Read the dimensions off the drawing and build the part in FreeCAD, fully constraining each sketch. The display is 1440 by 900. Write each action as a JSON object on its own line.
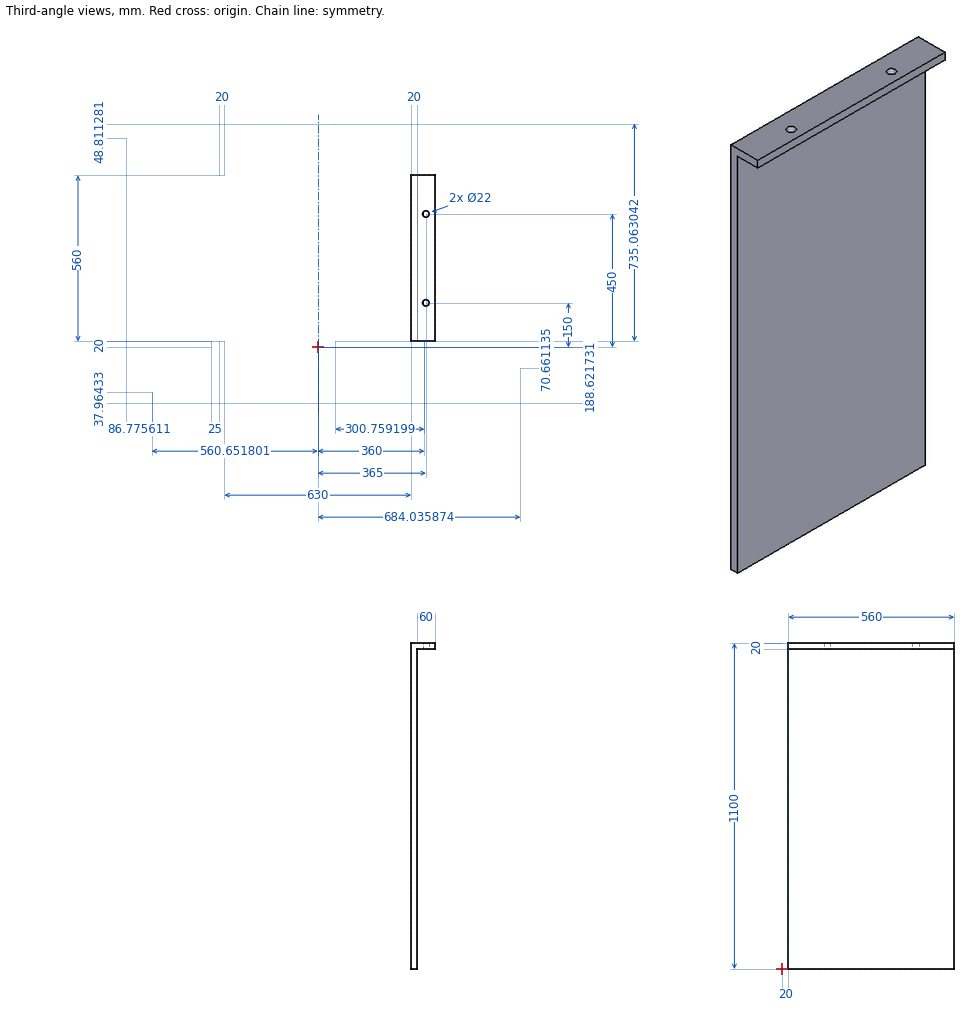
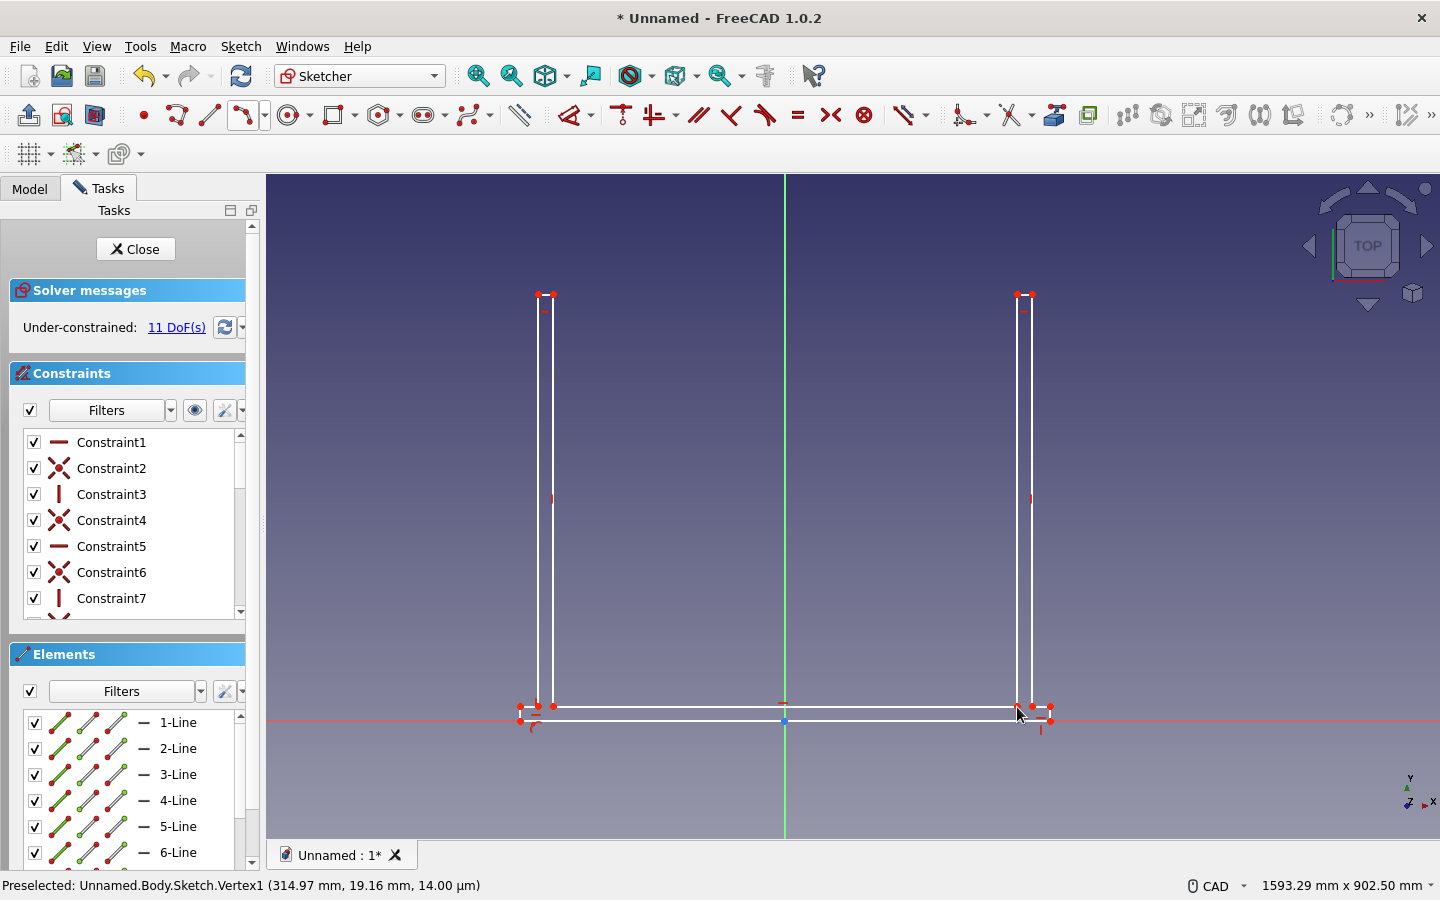
{"action": "left_click", "coordinate": [520, 707]}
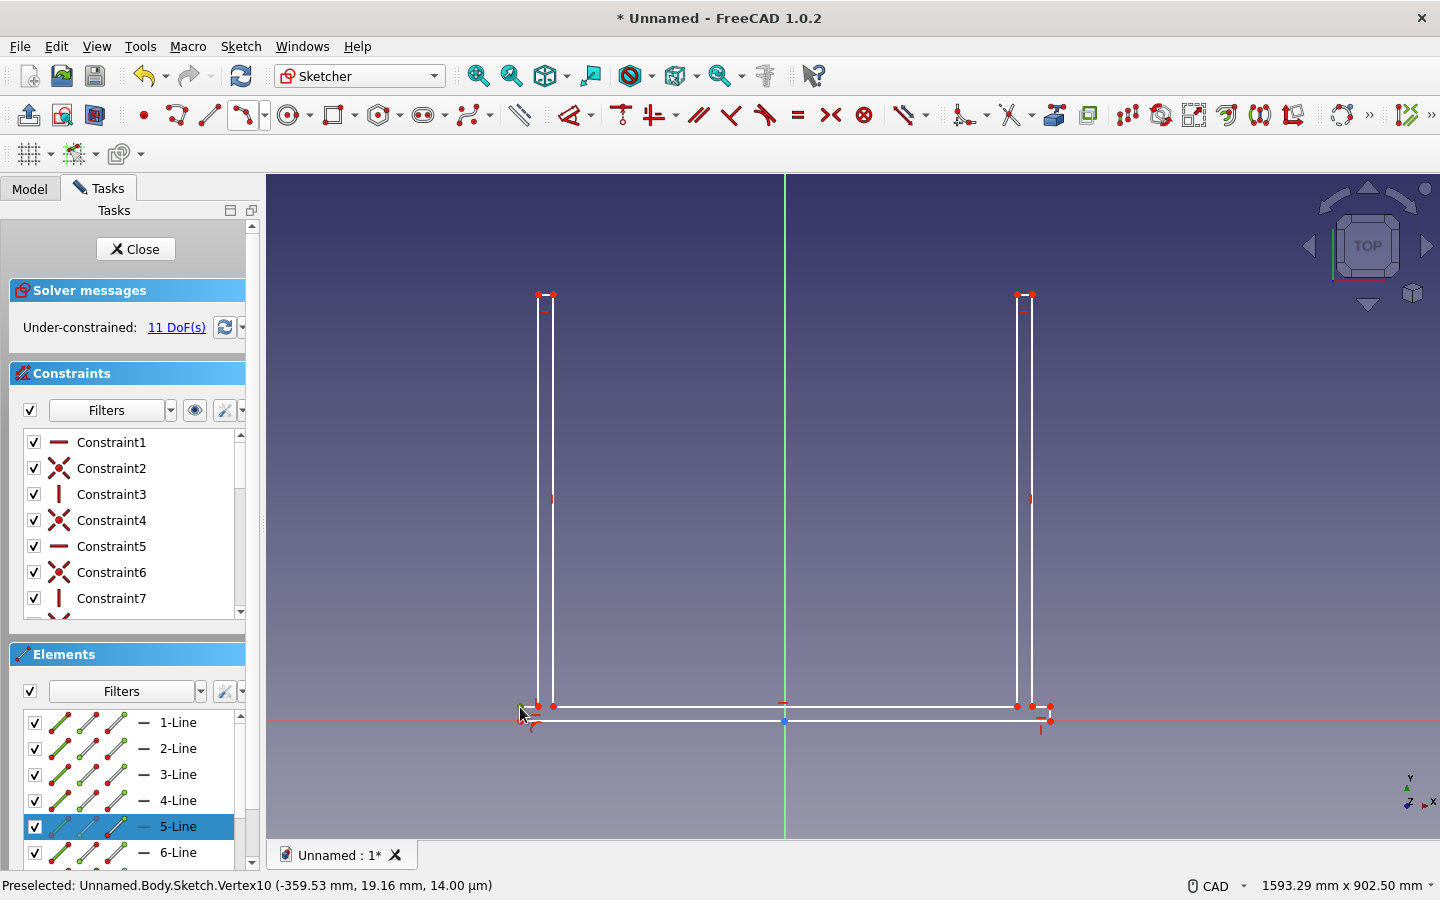
{"action": "left_click", "coordinate": [1050, 707]}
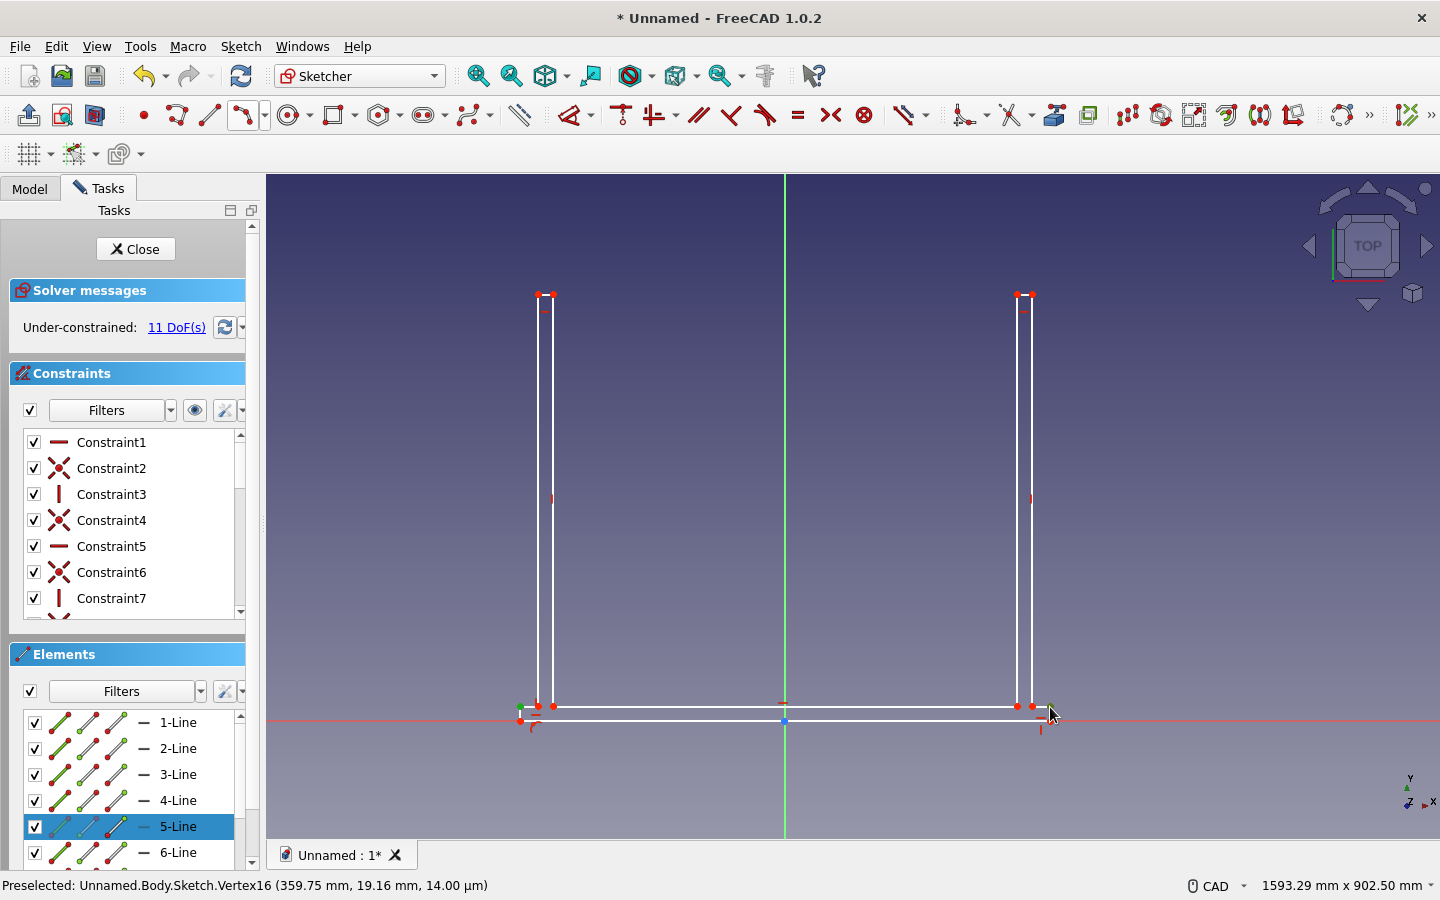
{"action": "left_click", "coordinate": [785, 768]}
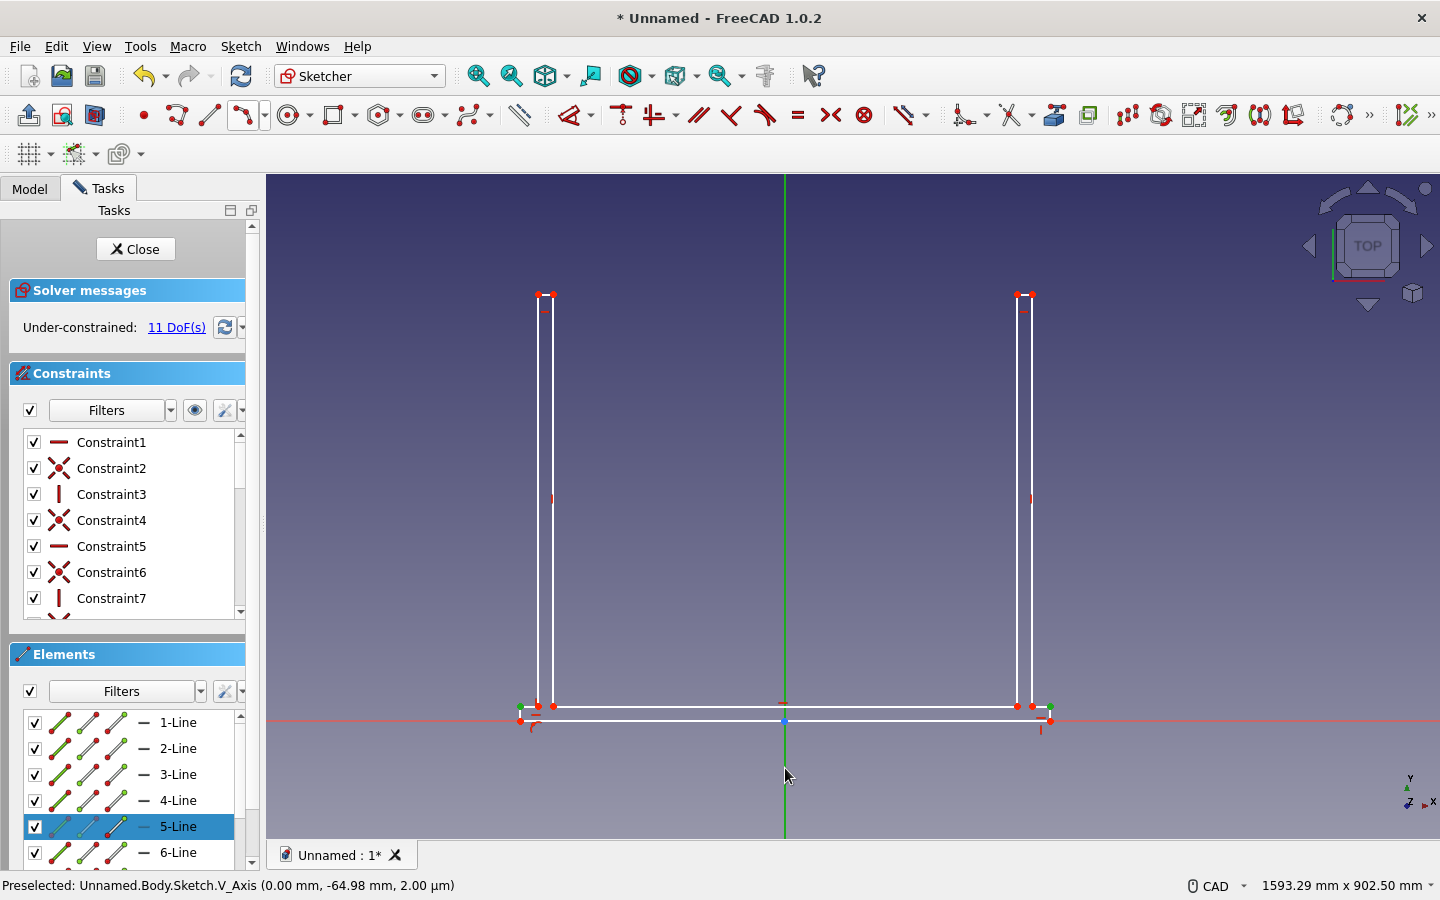
{"action": "key", "text": "s"}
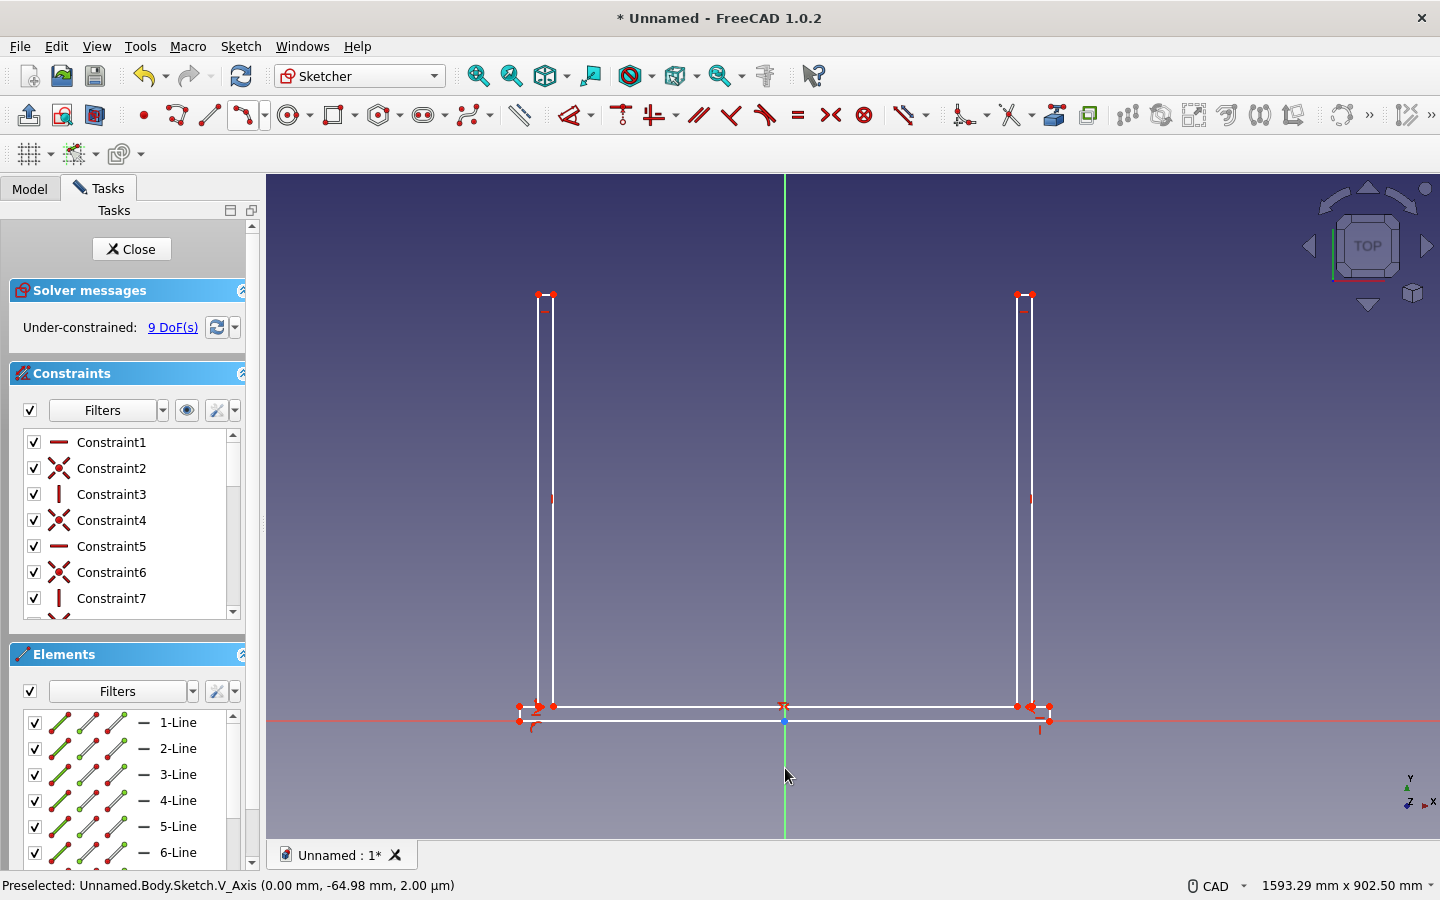
{"action": "left_click", "coordinate": [538, 295]}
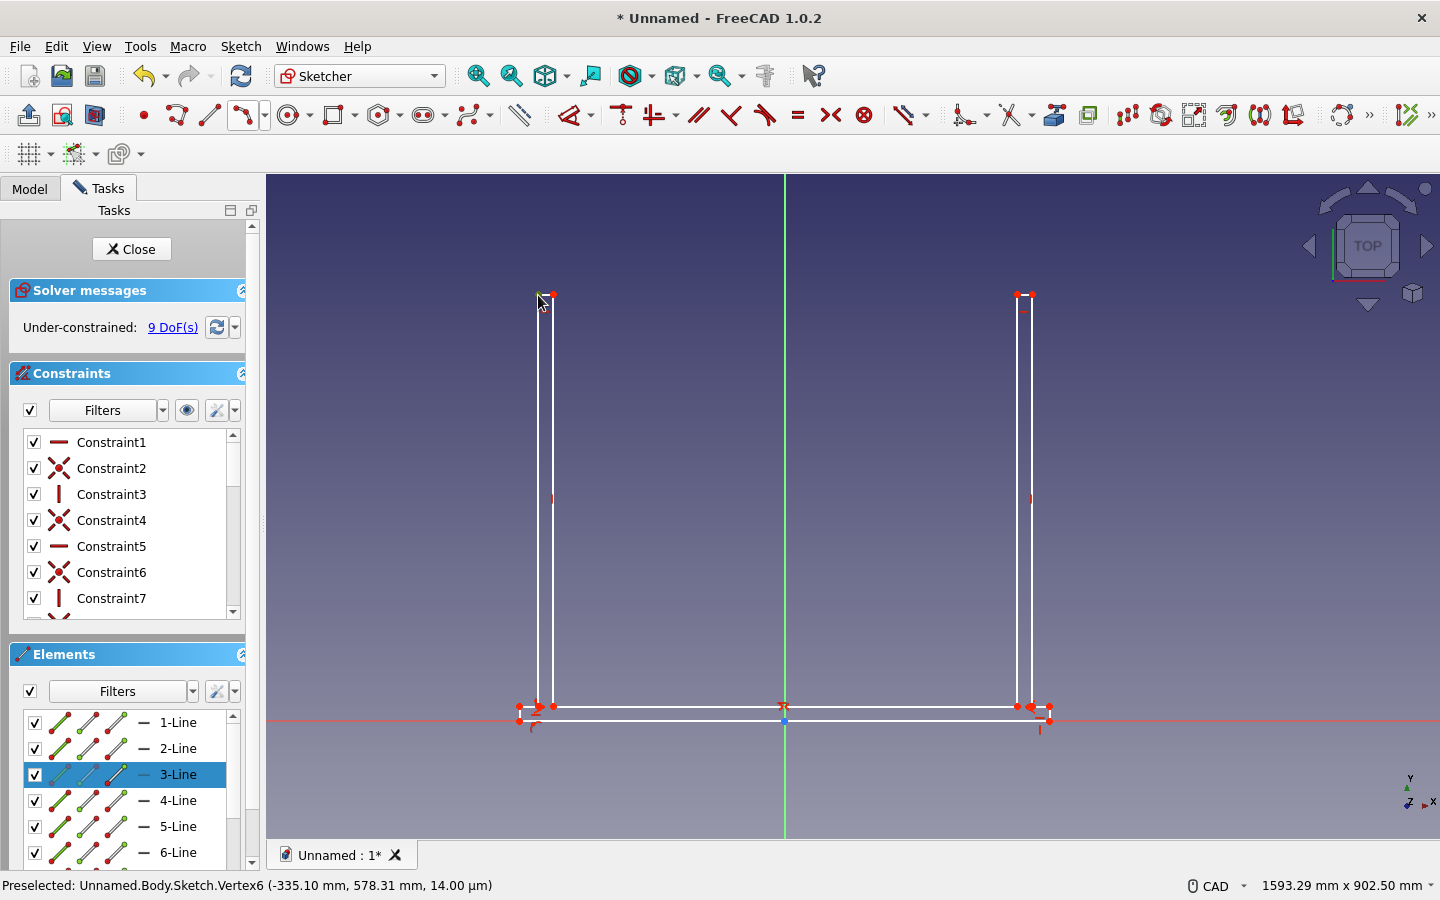
{"action": "left_click", "coordinate": [1032, 295]}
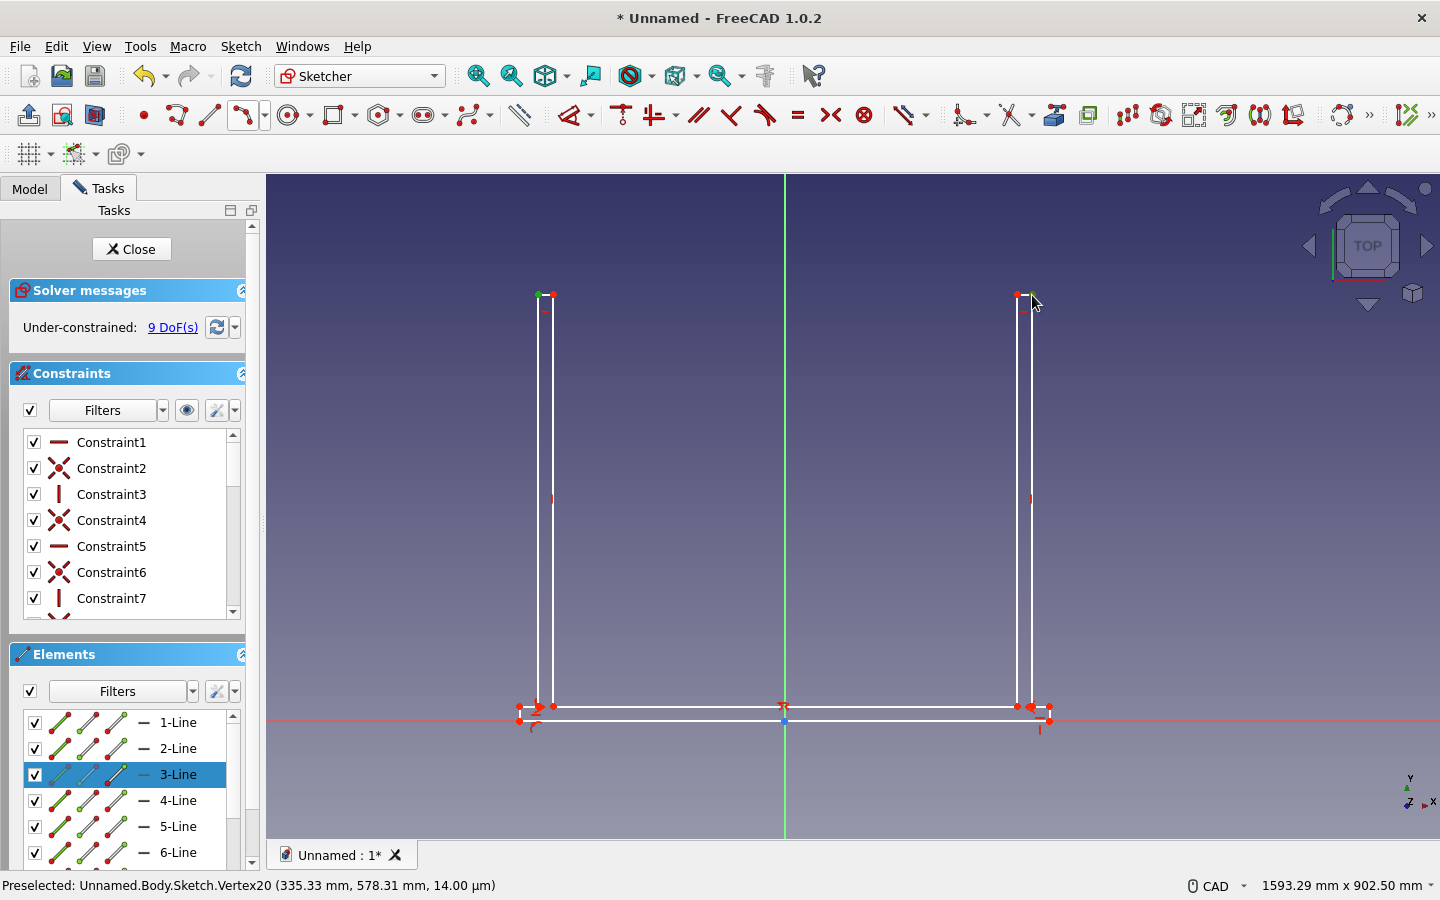
{"action": "left_click", "coordinate": [785, 768]}